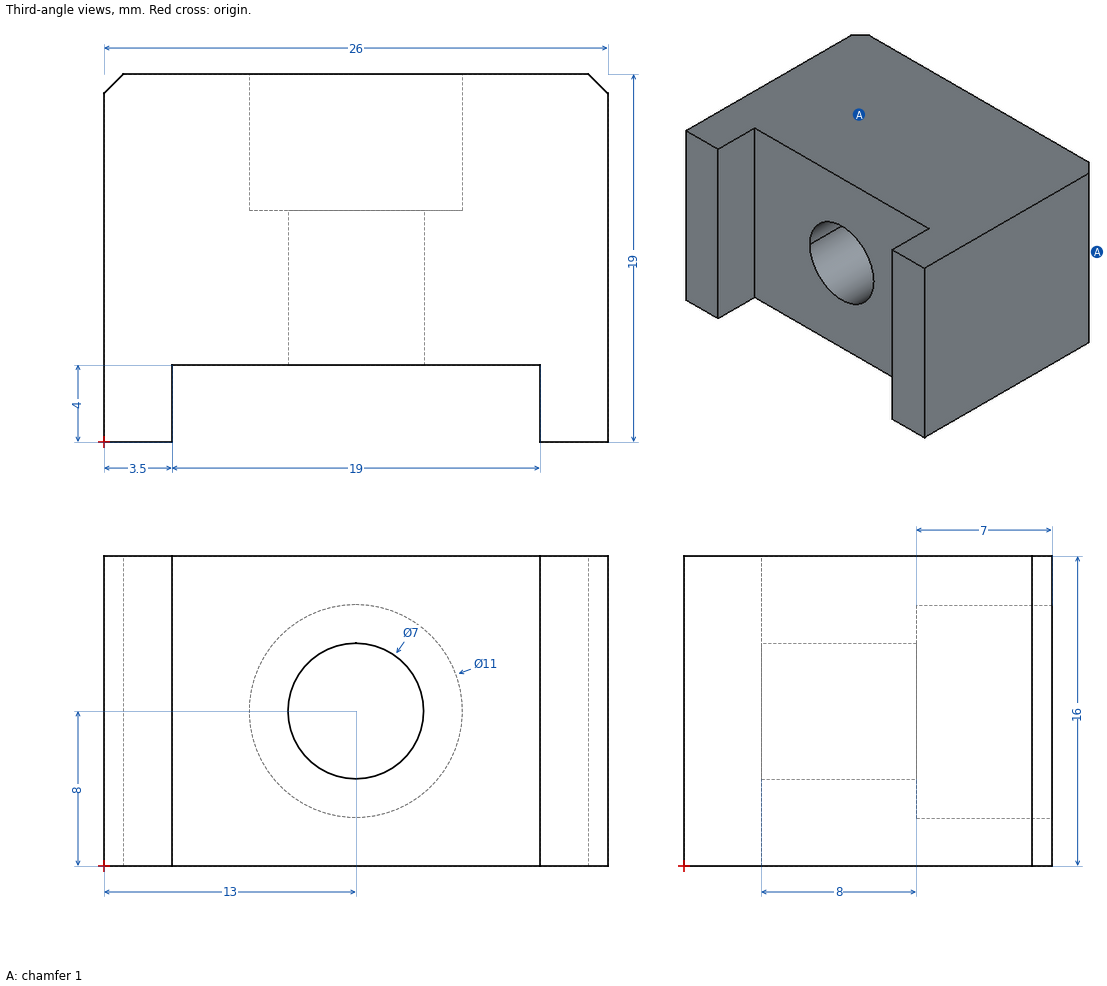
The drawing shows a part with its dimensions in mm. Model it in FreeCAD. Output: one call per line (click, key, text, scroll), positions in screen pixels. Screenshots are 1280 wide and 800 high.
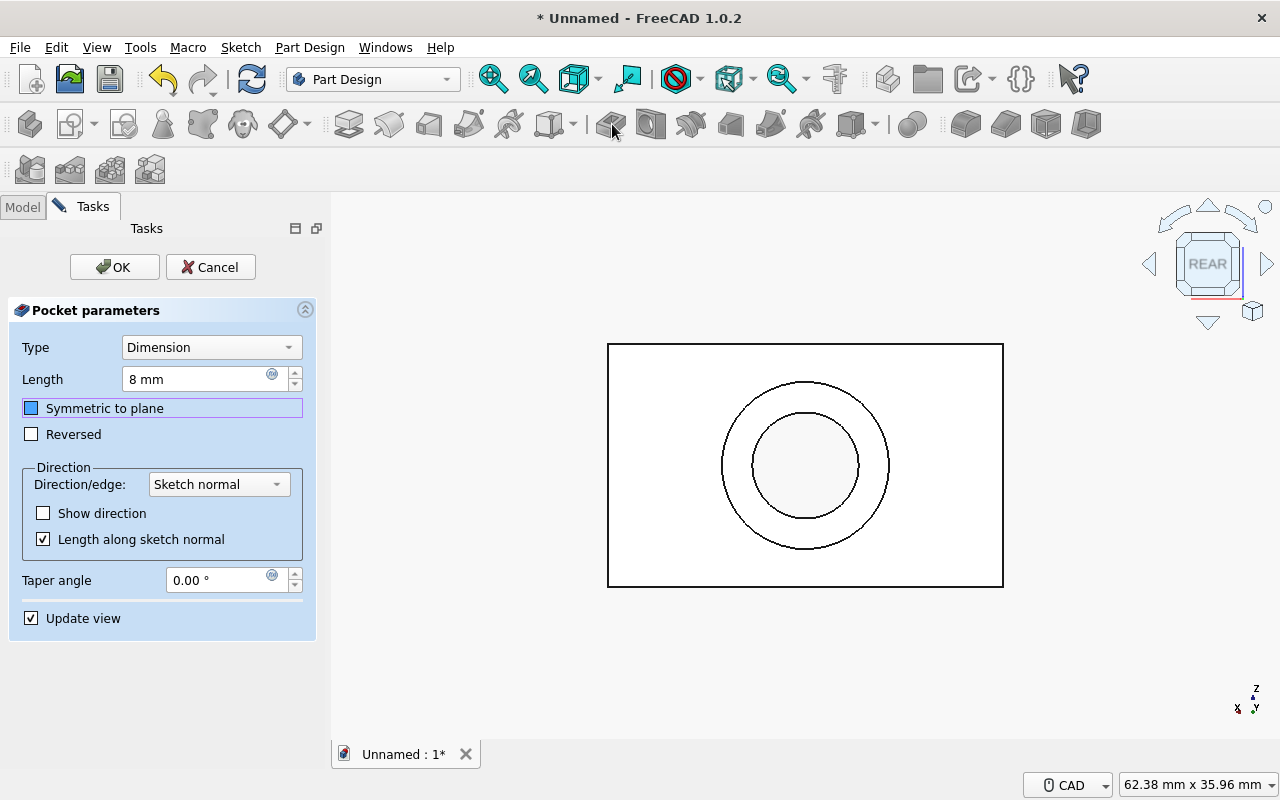
click(115, 267)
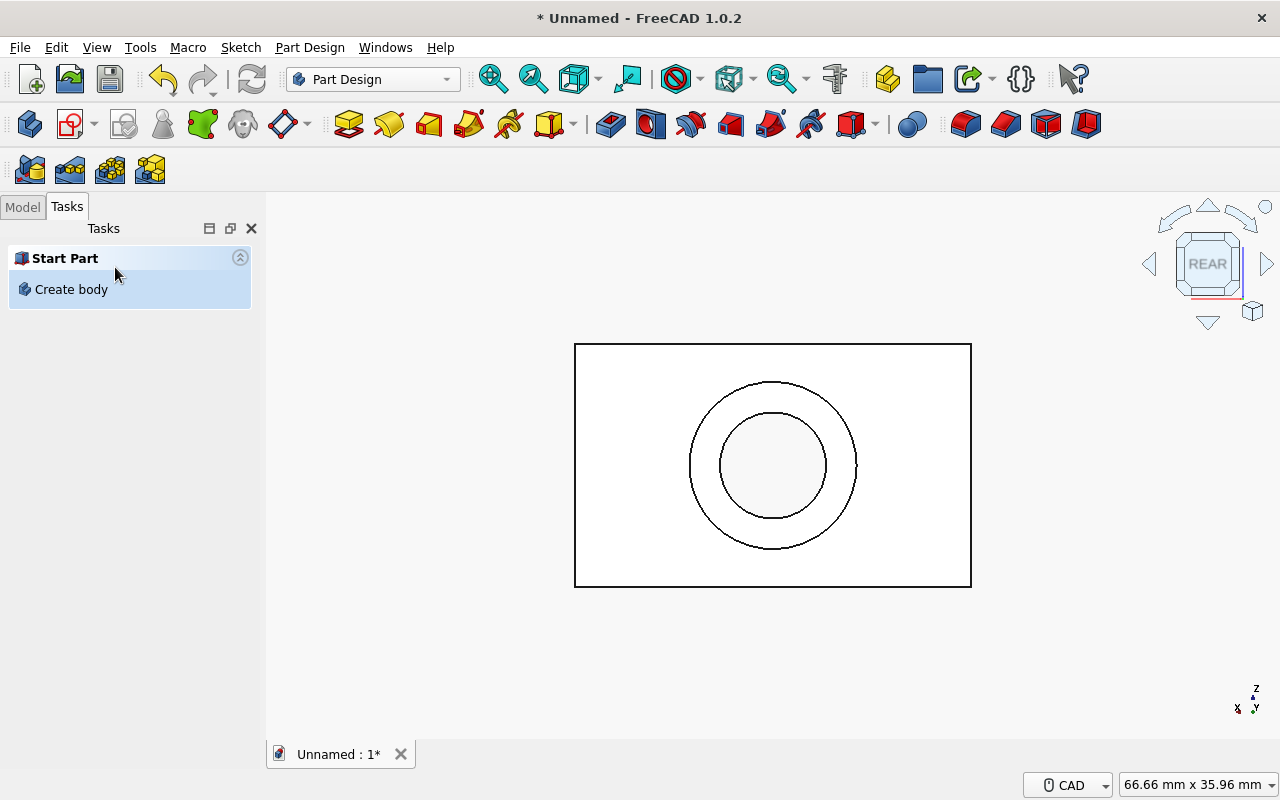
key(v)
key(f)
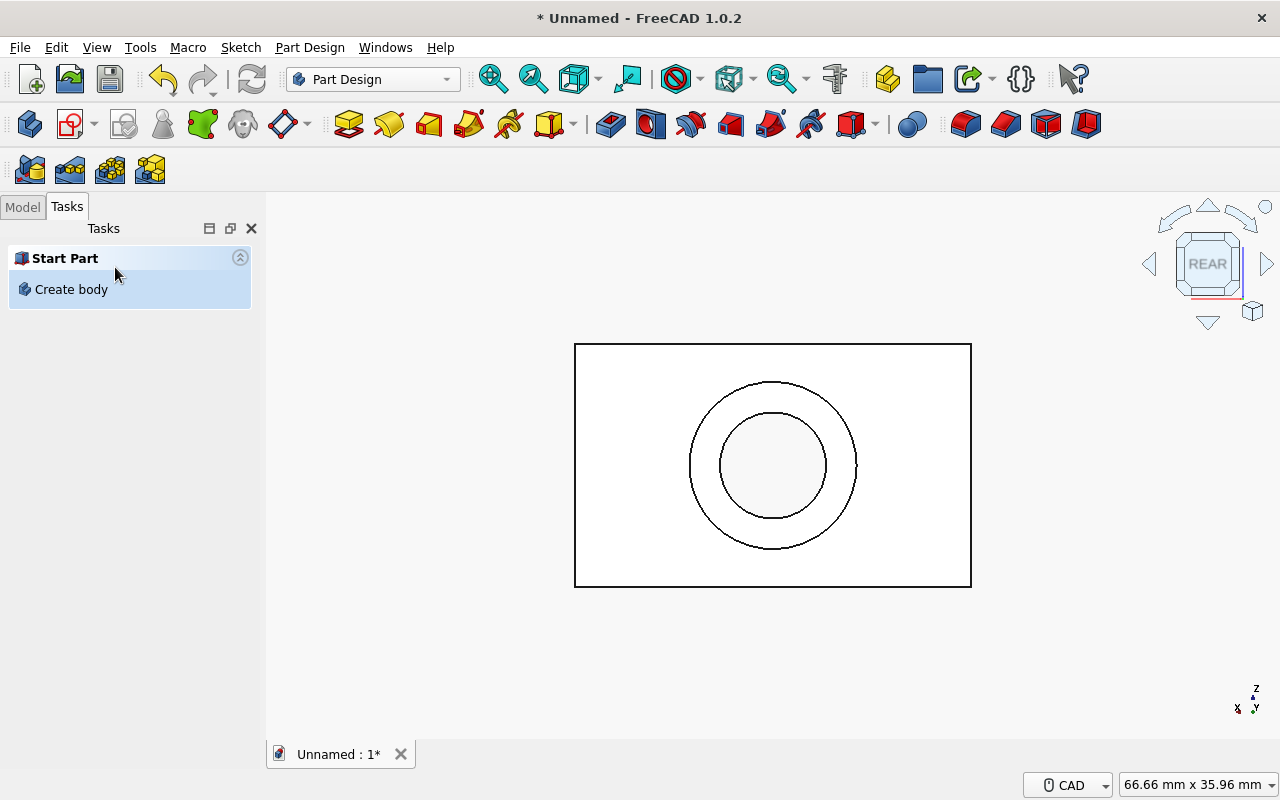
click(971, 464)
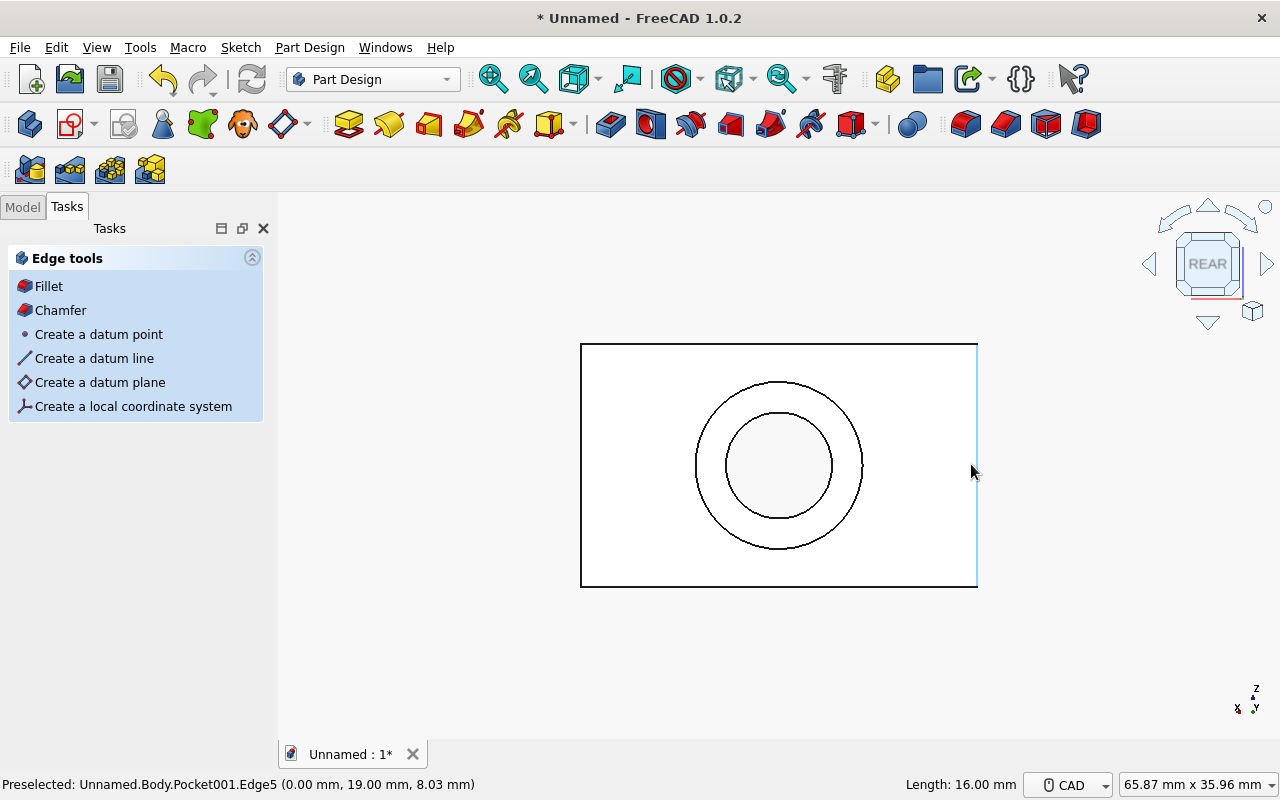
key(0)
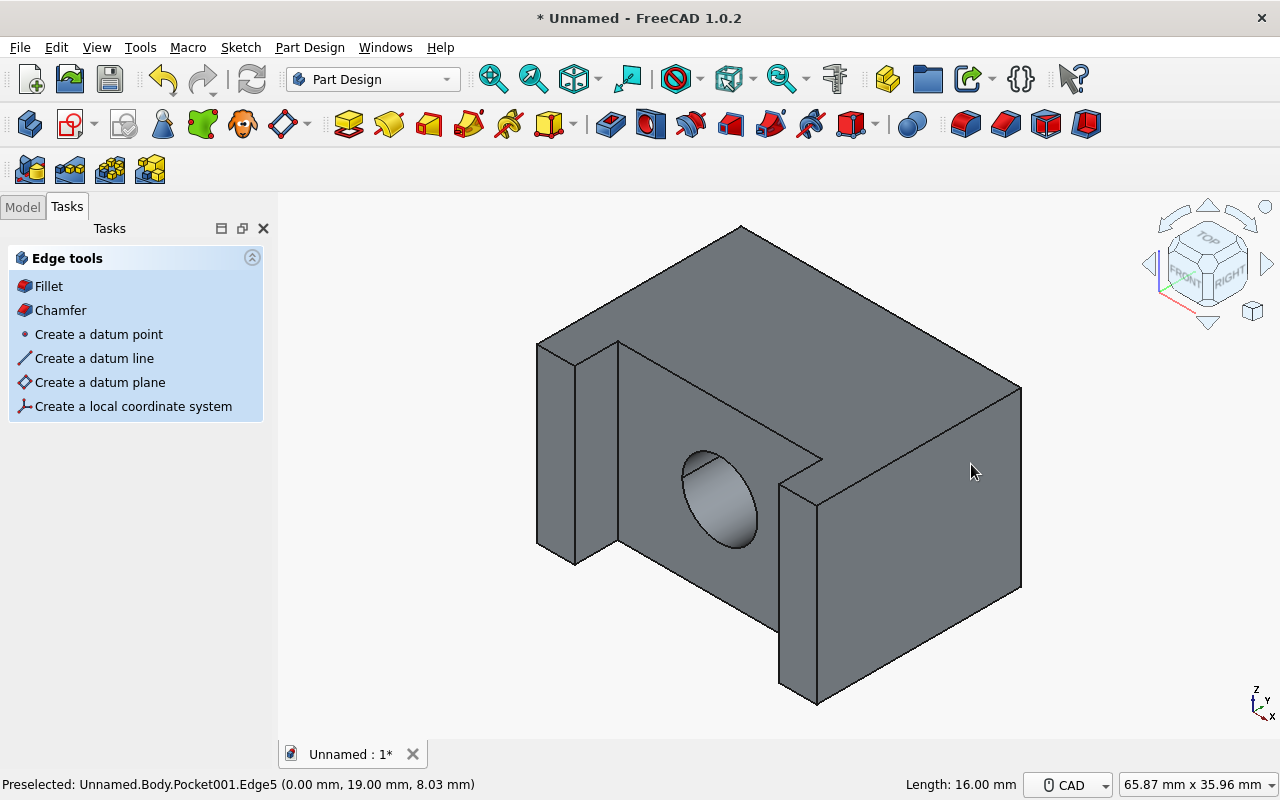
key(2)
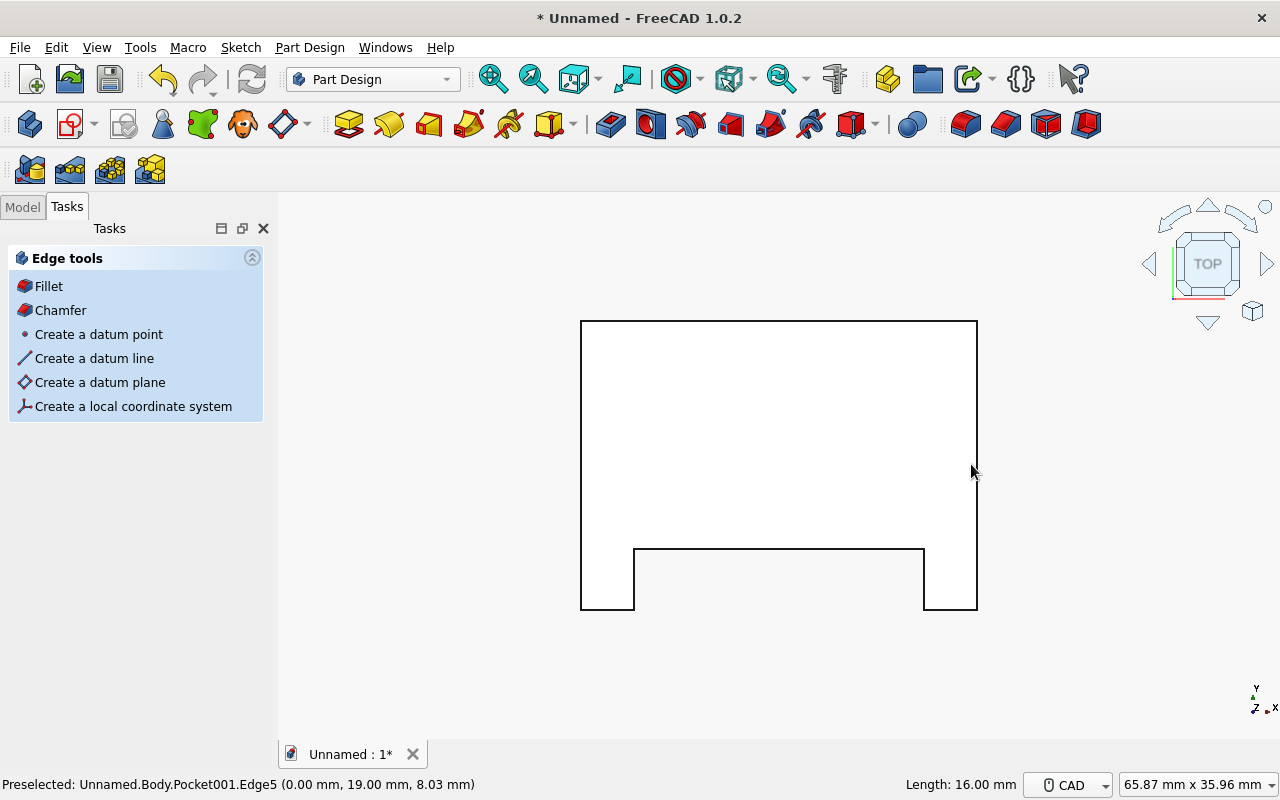
key(1)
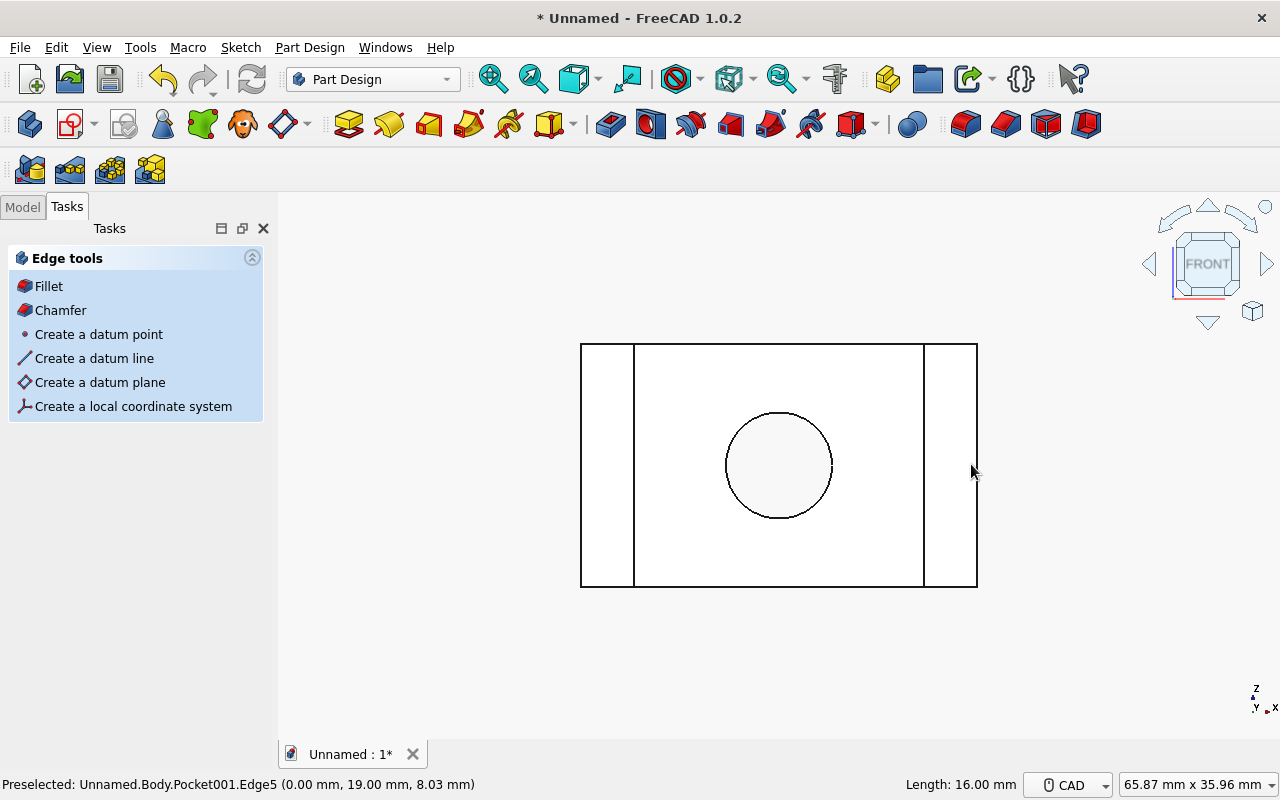
click(494, 80)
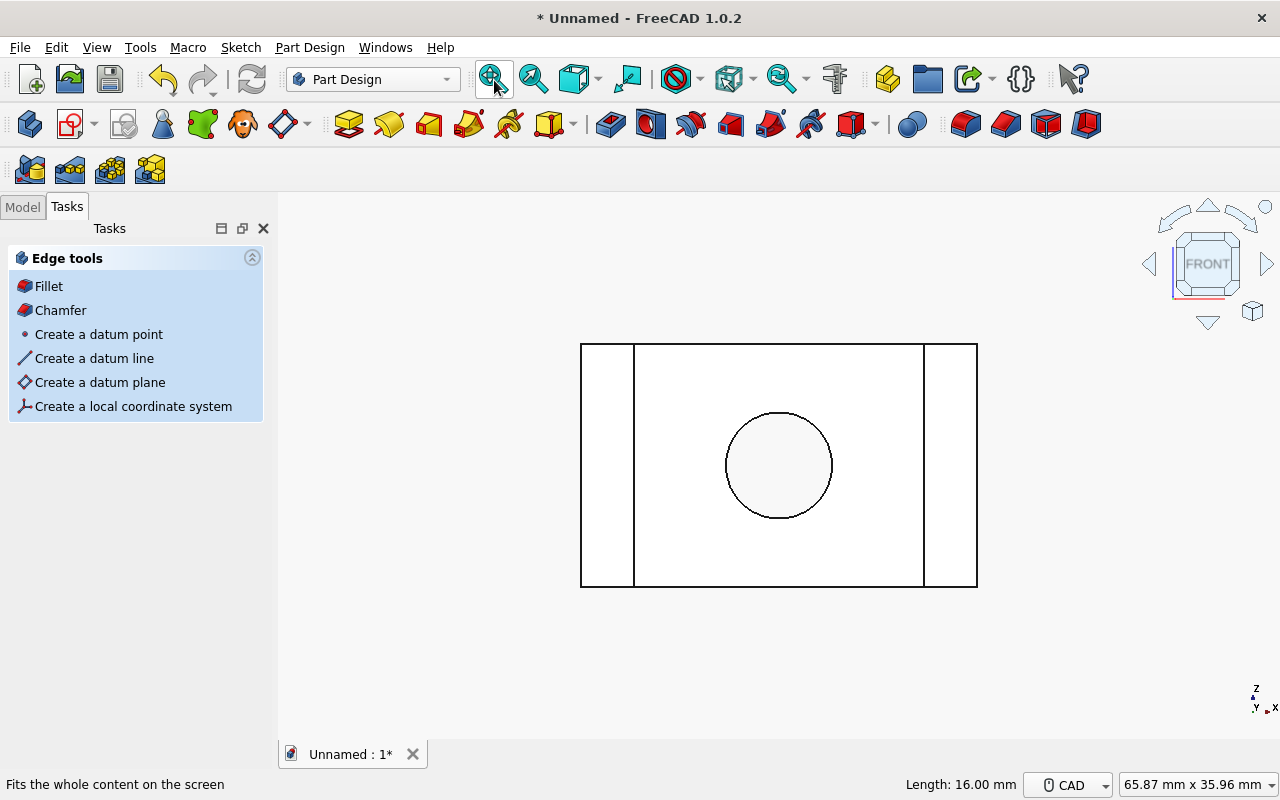
key(3)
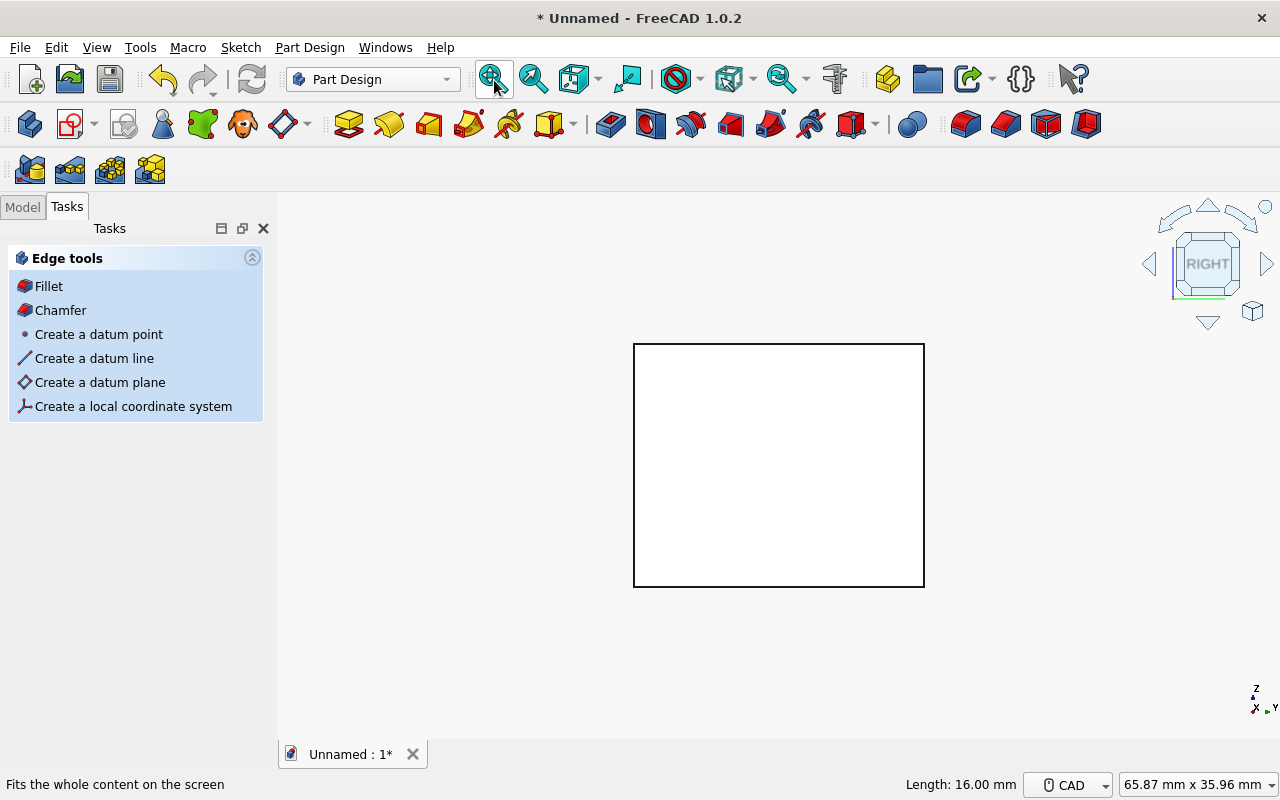
key(v)
key(f)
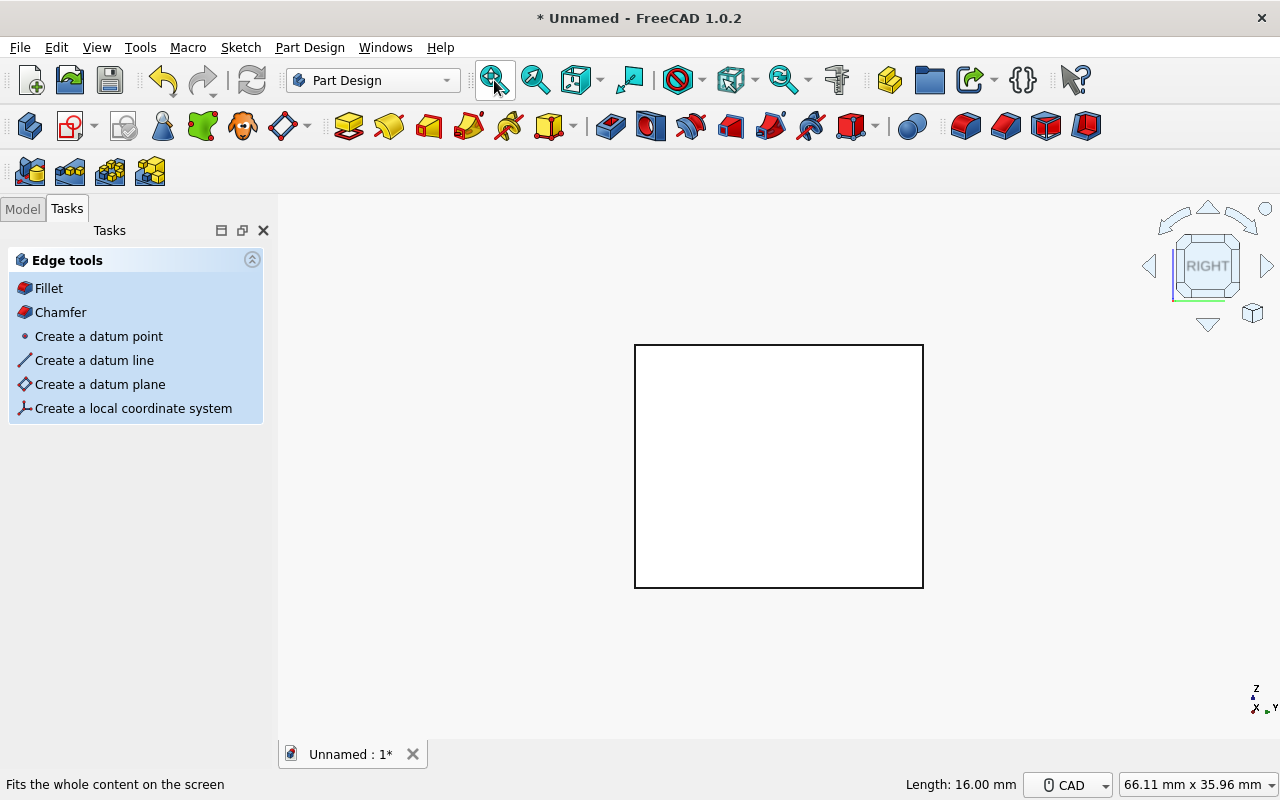
click(923, 465, ctrl)